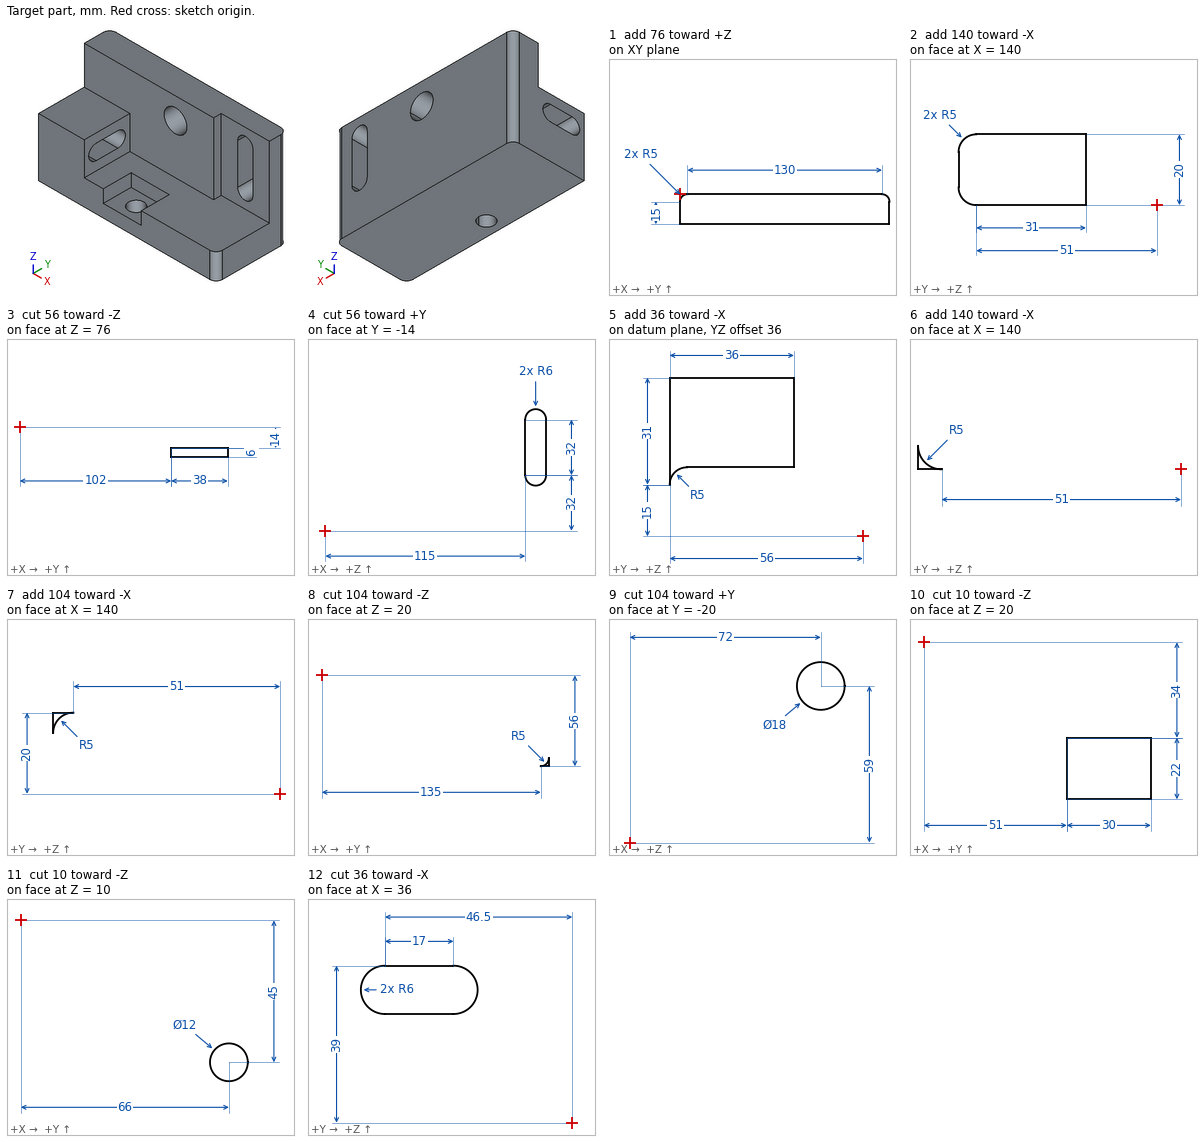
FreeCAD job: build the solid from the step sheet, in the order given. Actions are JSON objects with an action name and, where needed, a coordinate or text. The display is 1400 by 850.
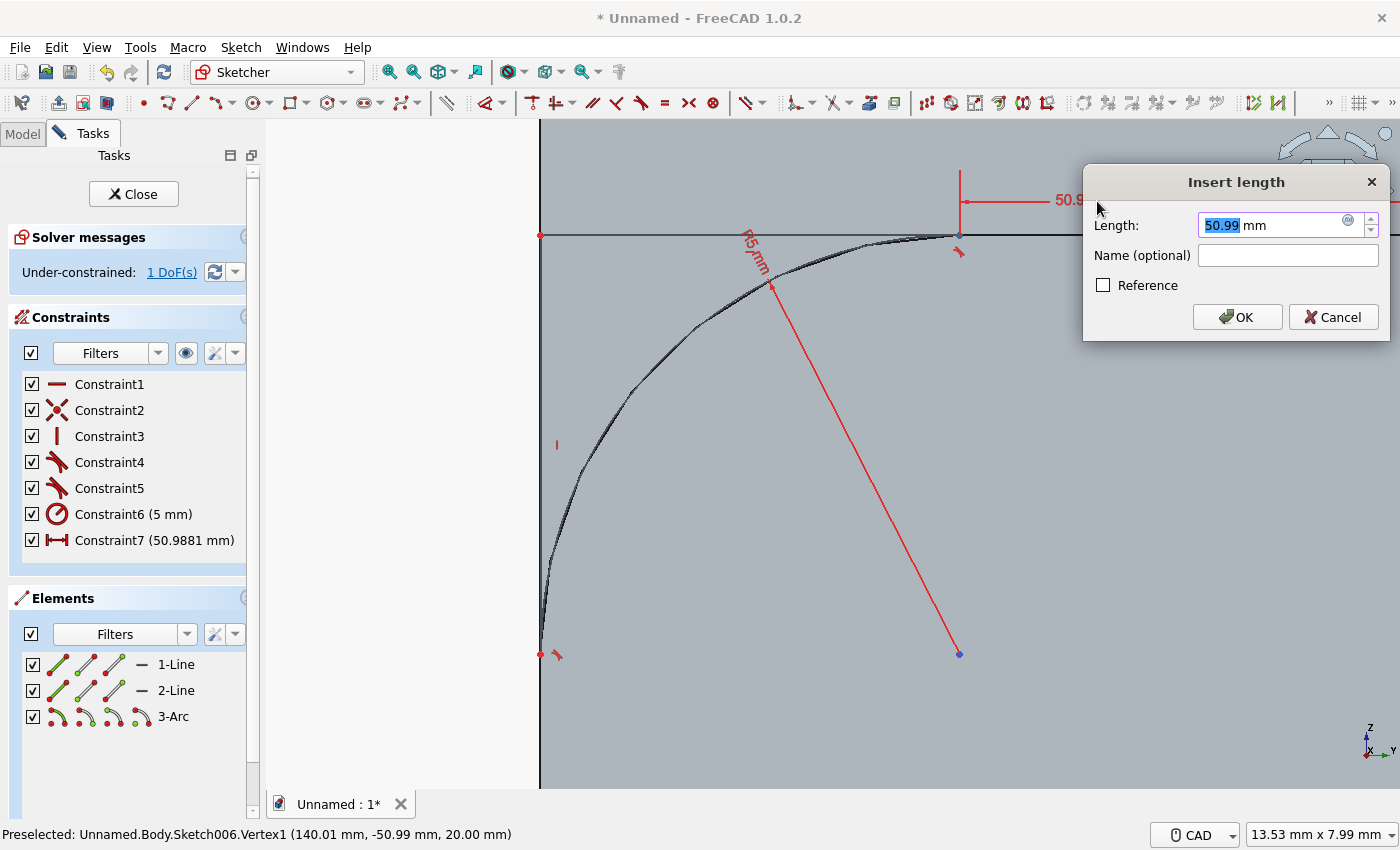
{"action": "type", "text": "51"}
{"action": "key", "text": "Return"}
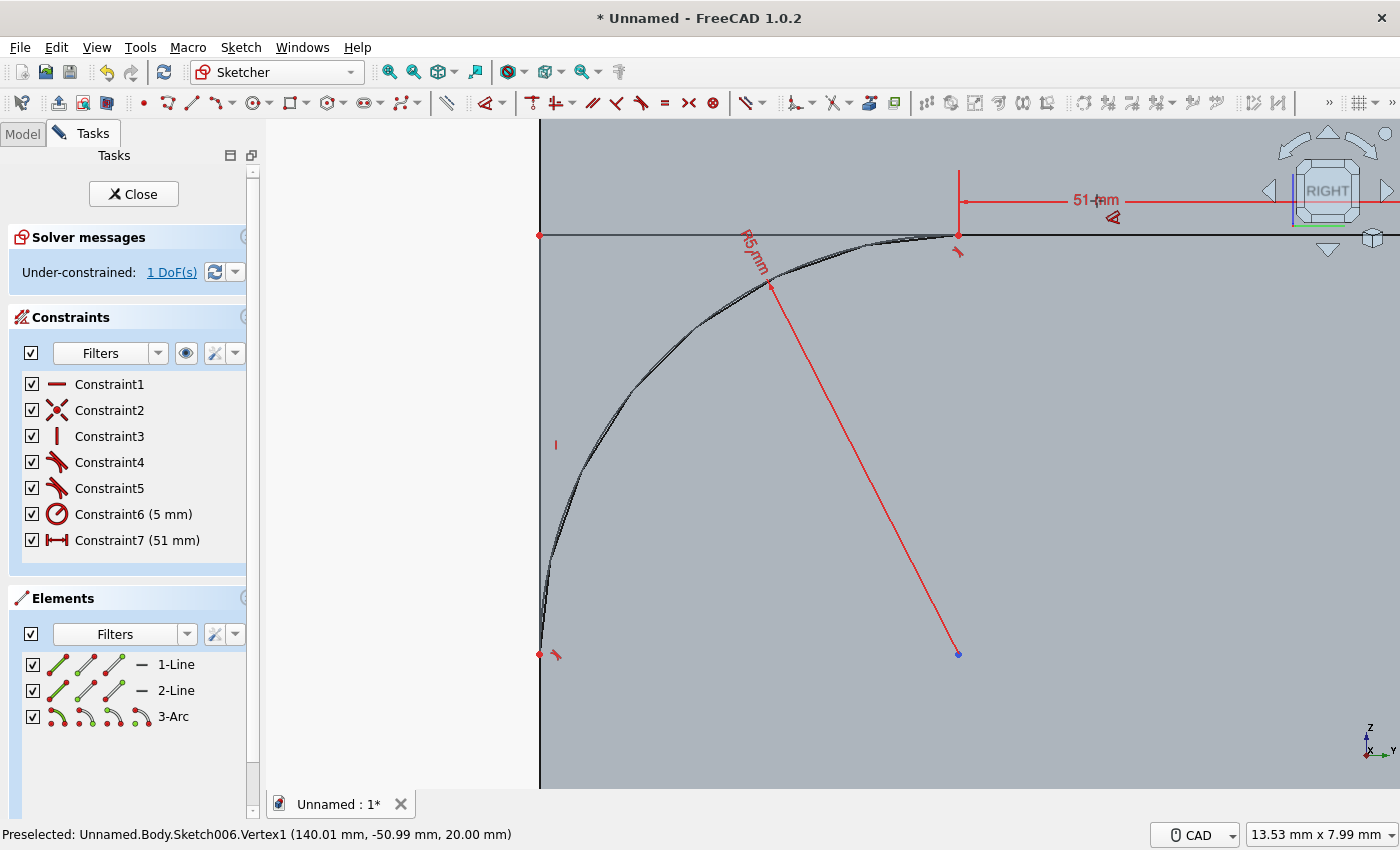
{"action": "left_click", "coordinate": [959, 235]}
{"action": "left_click", "coordinate": [925, 498]}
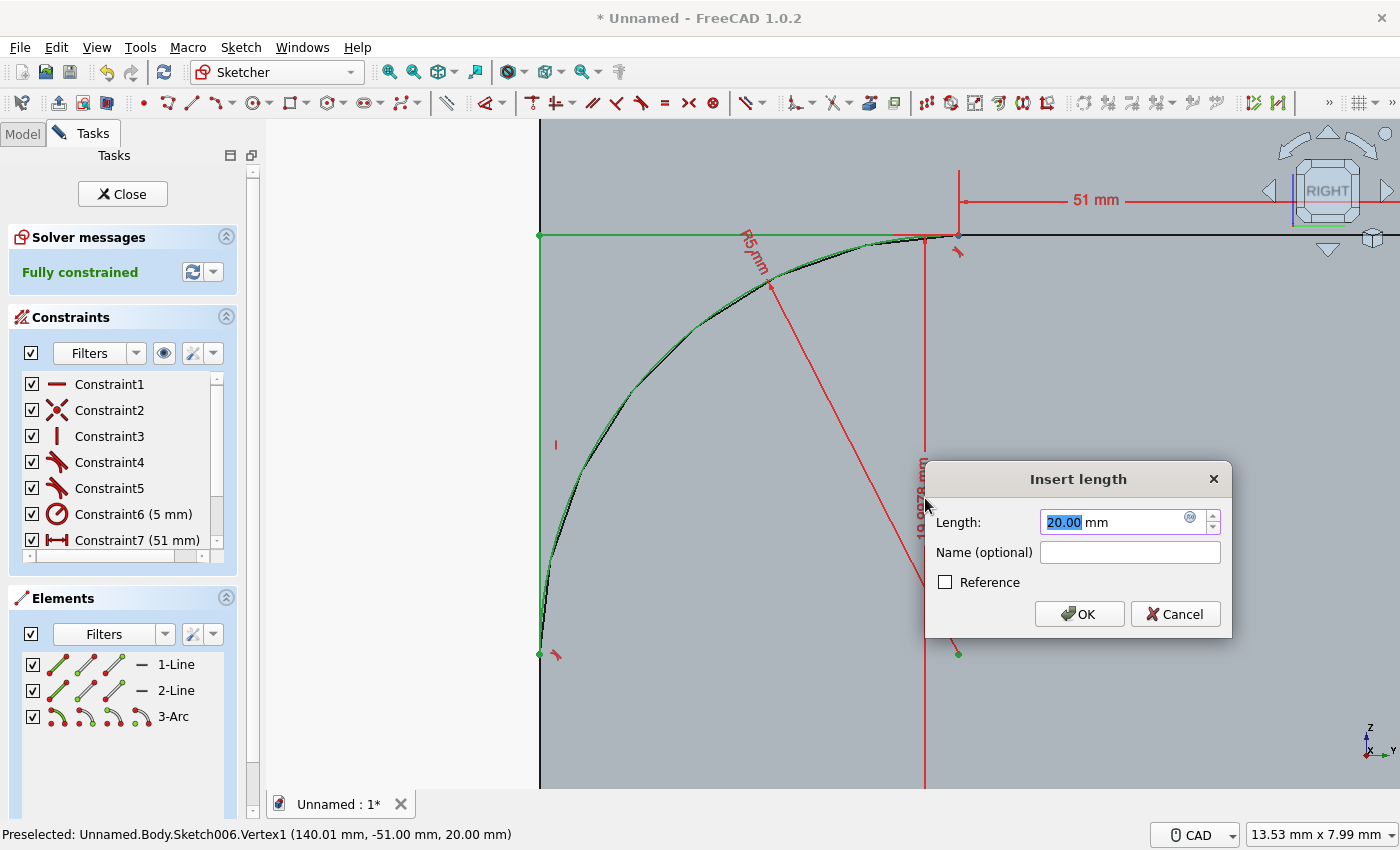
{"action": "type", "text": "20"}
{"action": "key", "text": "Return"}
{"action": "key", "text": "Escape"}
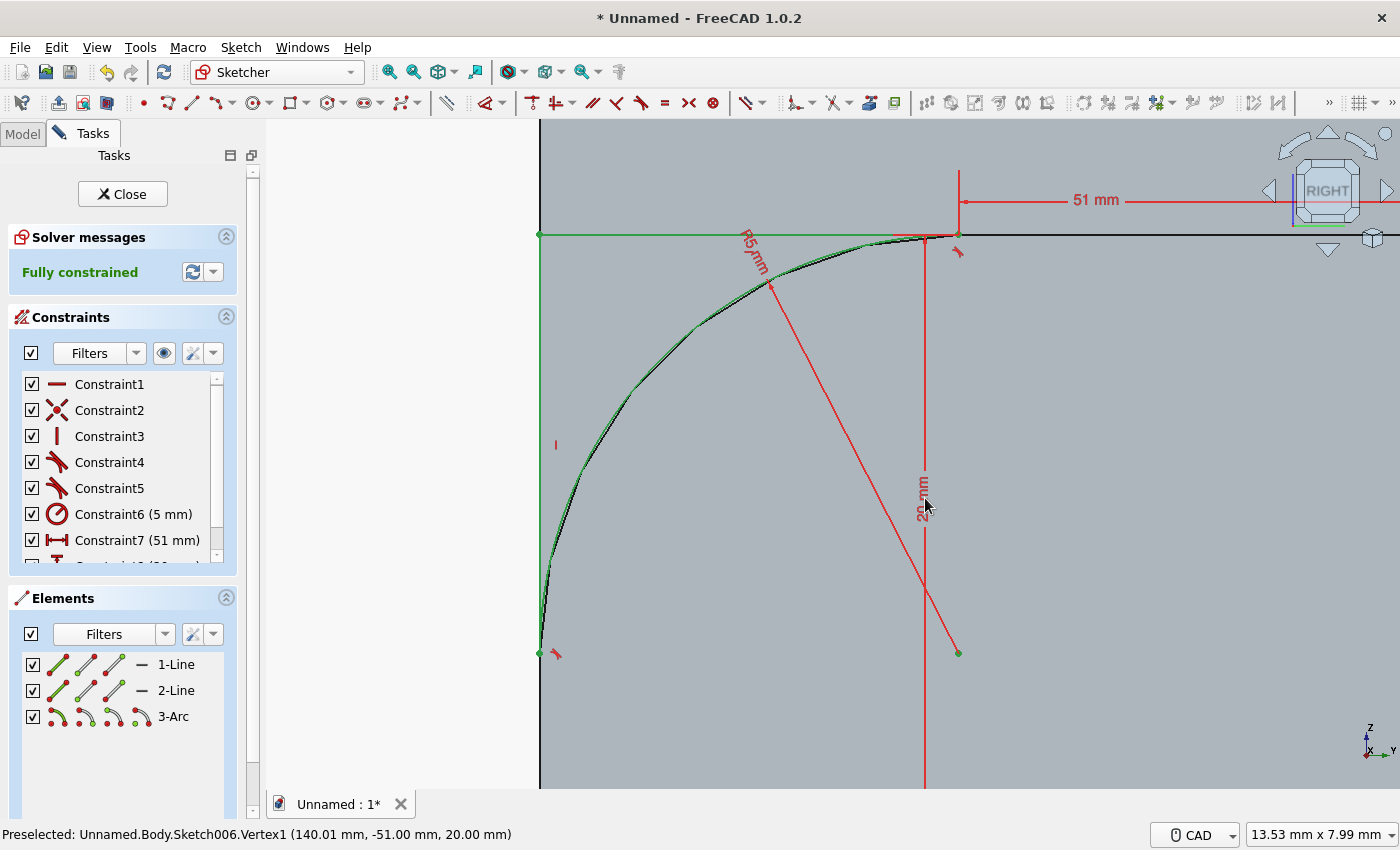
{"action": "left_click", "coordinate": [123, 194]}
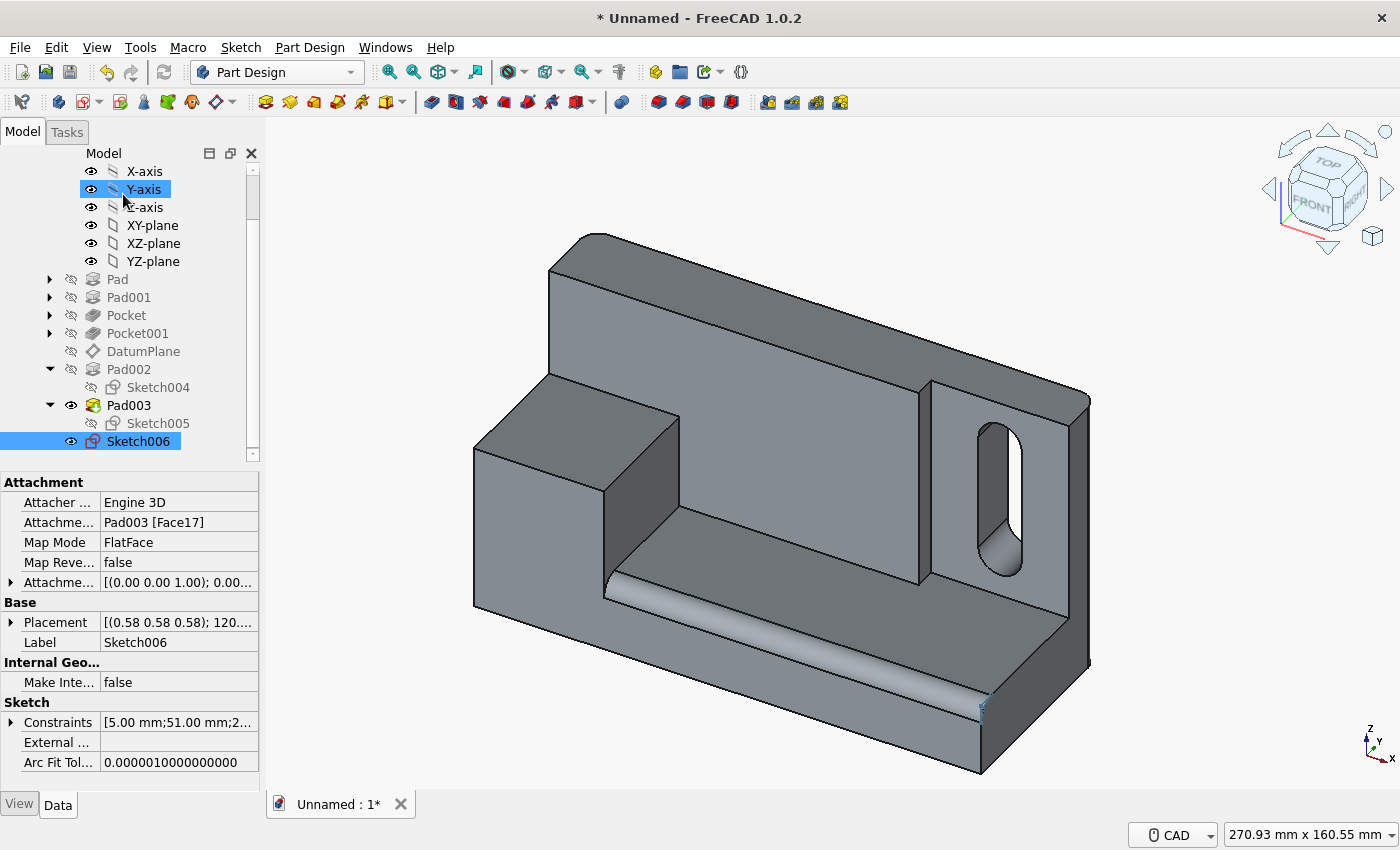
{"action": "left_click", "coordinate": [266, 102]}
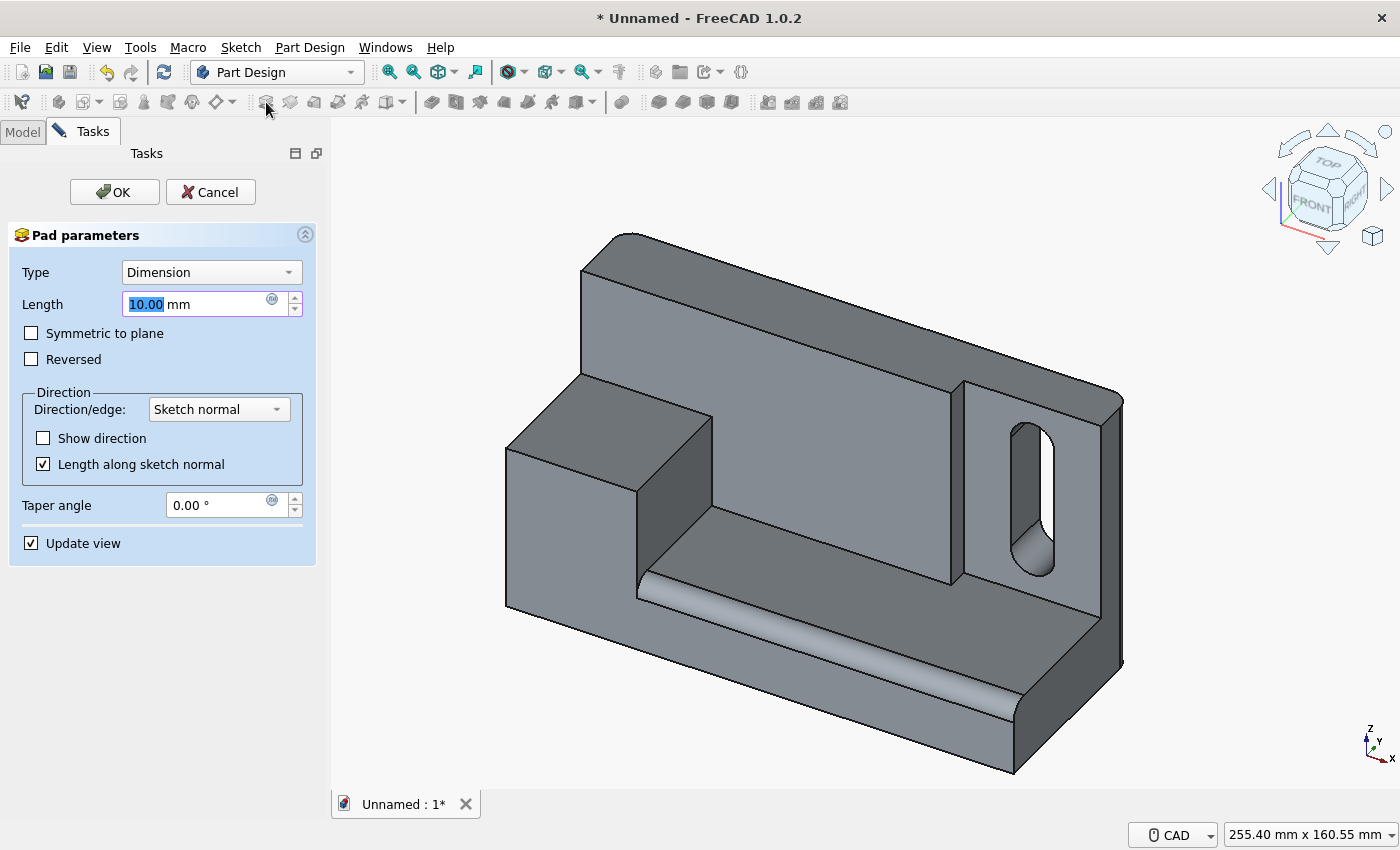
{"action": "type", "text": "104"}
{"action": "key", "text": "Tab"}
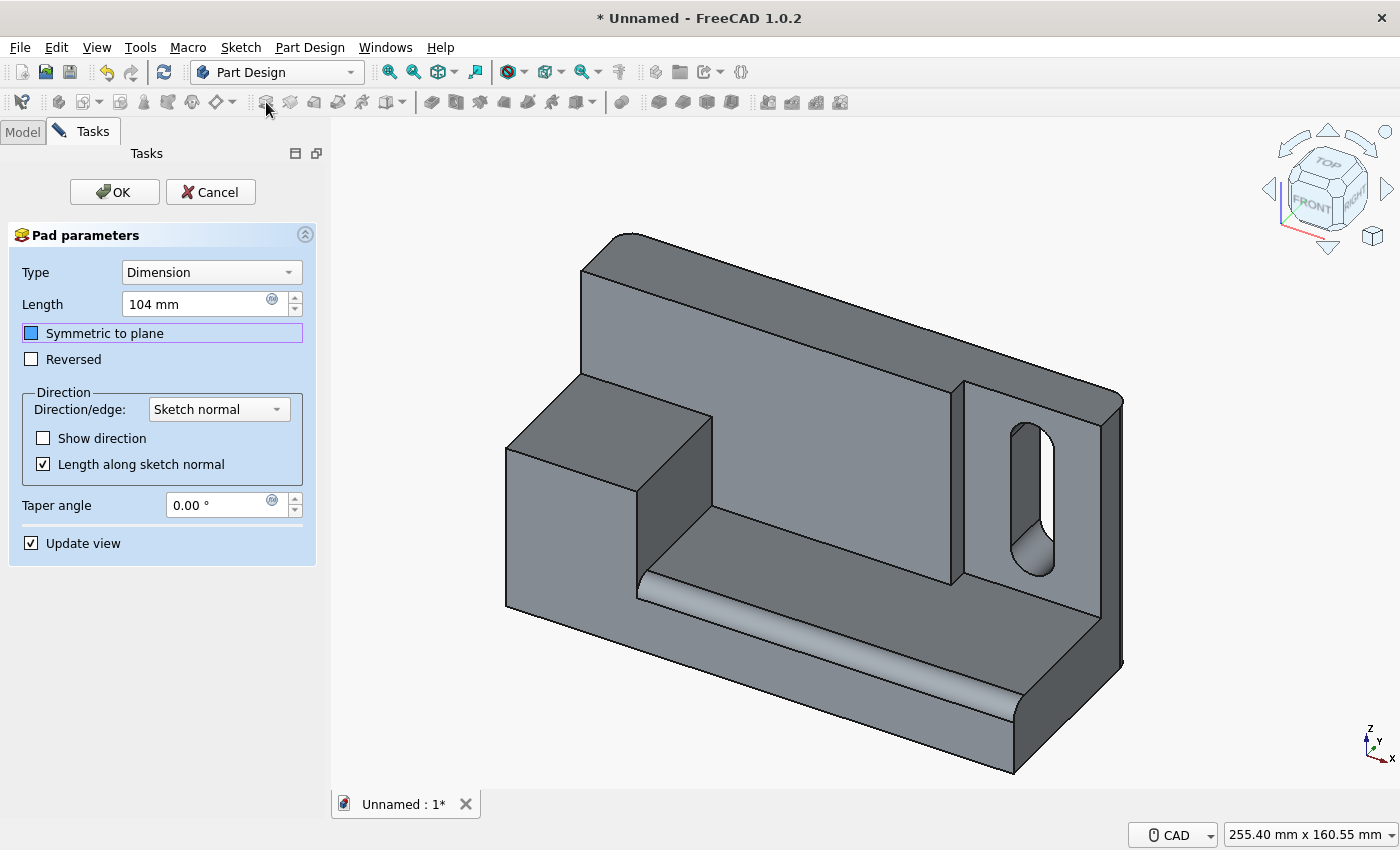
{"action": "left_click", "coordinate": [30, 359]}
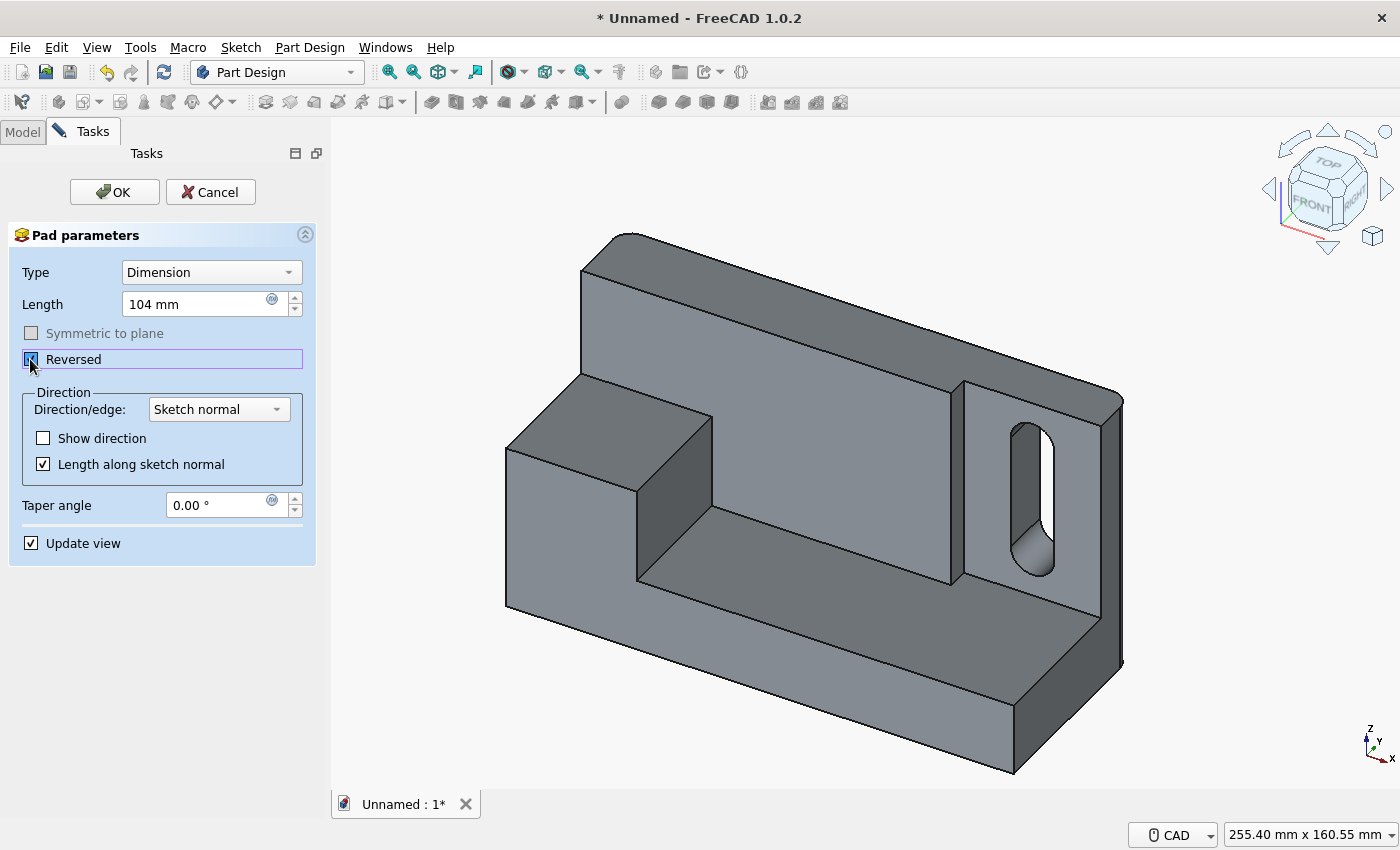
{"action": "left_click", "coordinate": [115, 192]}